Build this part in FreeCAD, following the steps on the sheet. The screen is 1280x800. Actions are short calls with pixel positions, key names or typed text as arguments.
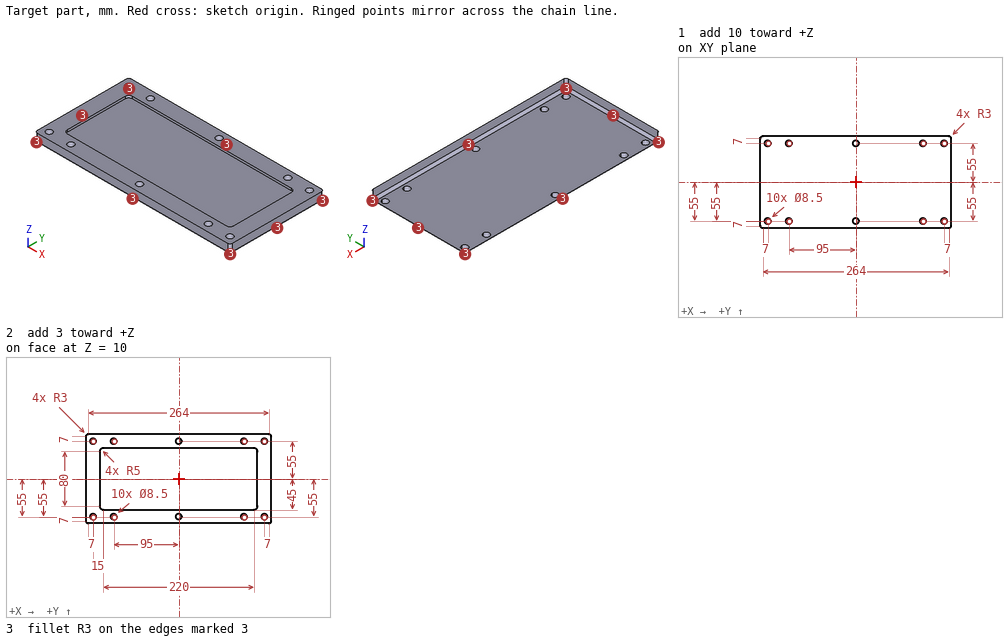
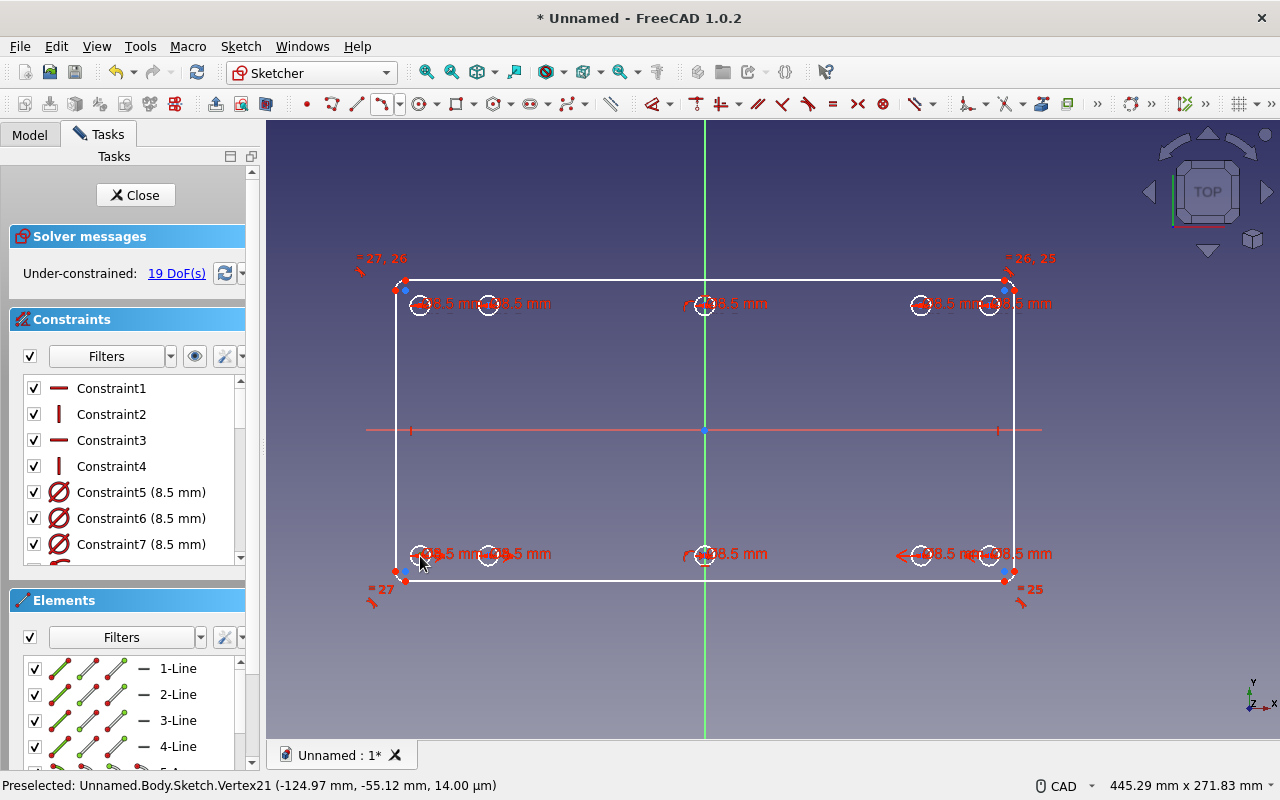
click(420, 306)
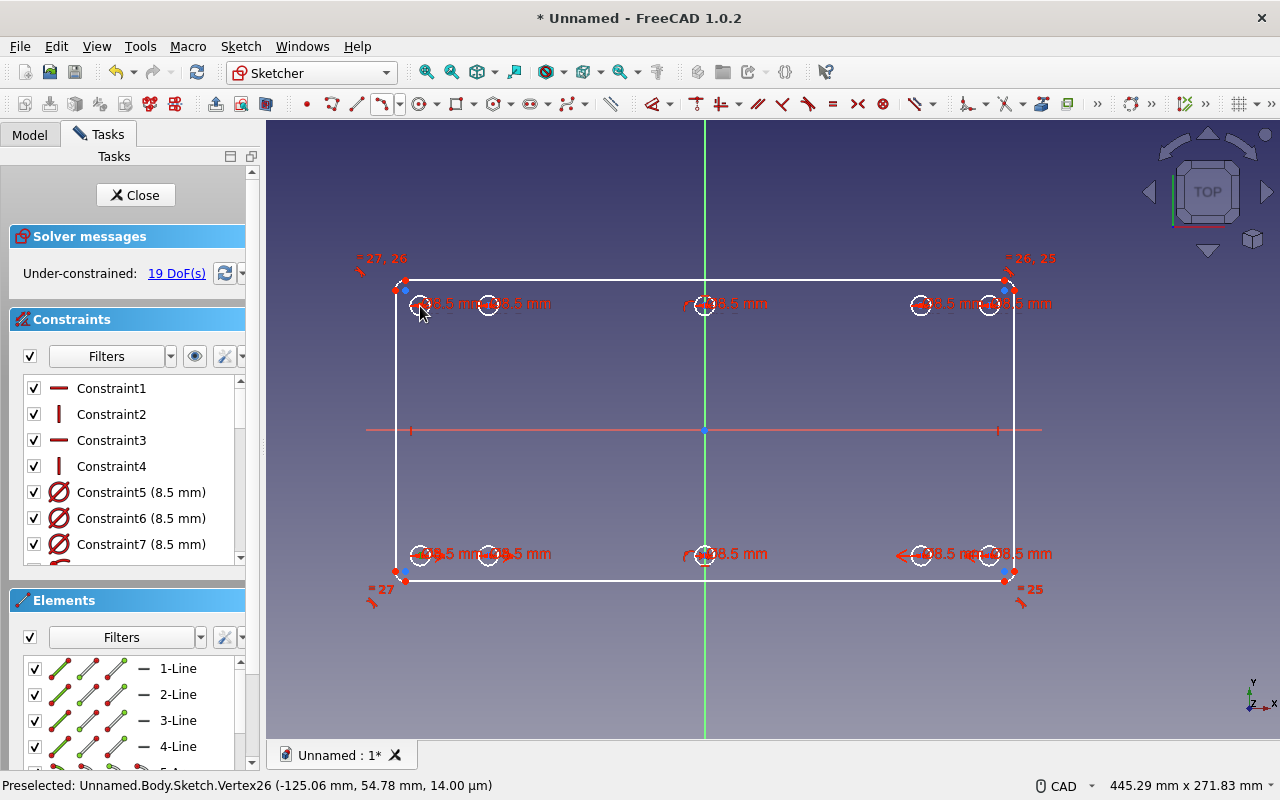
click(470, 430)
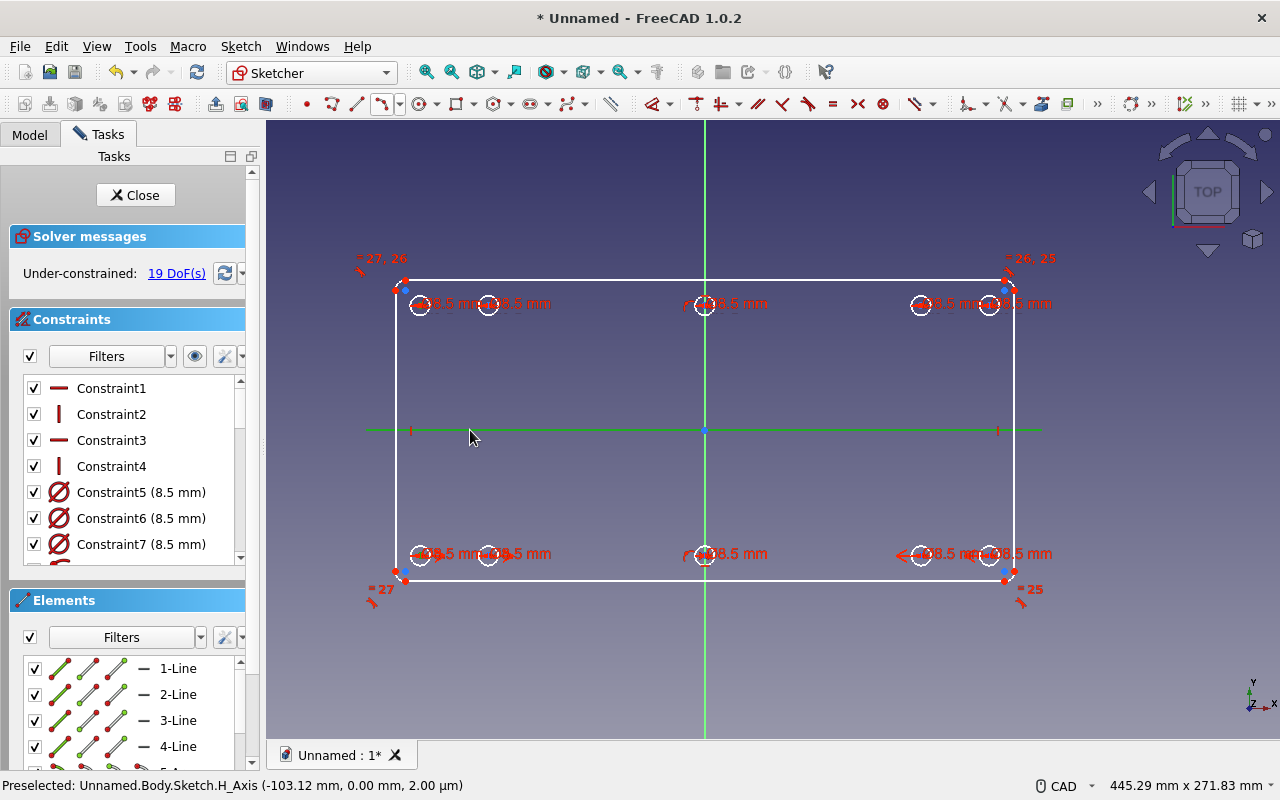
click(858, 104)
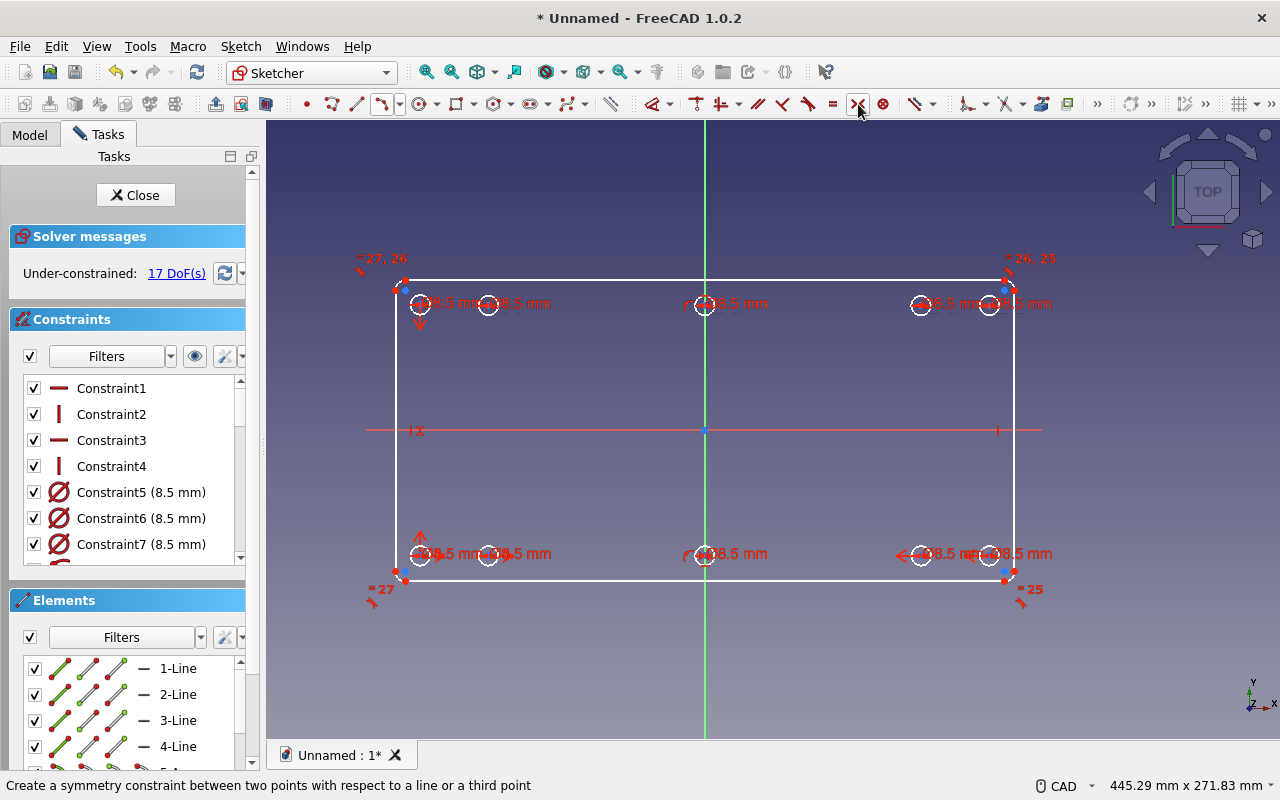
click(488, 556)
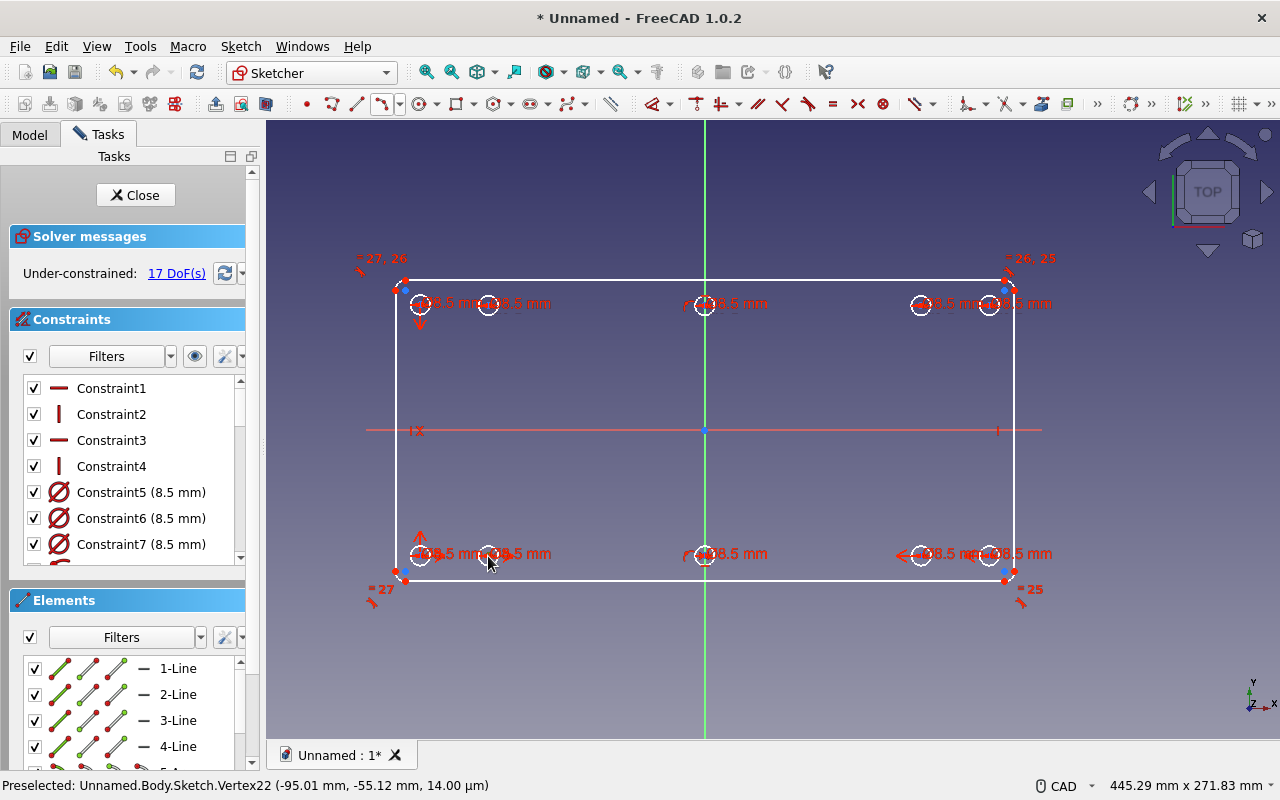
click(488, 306)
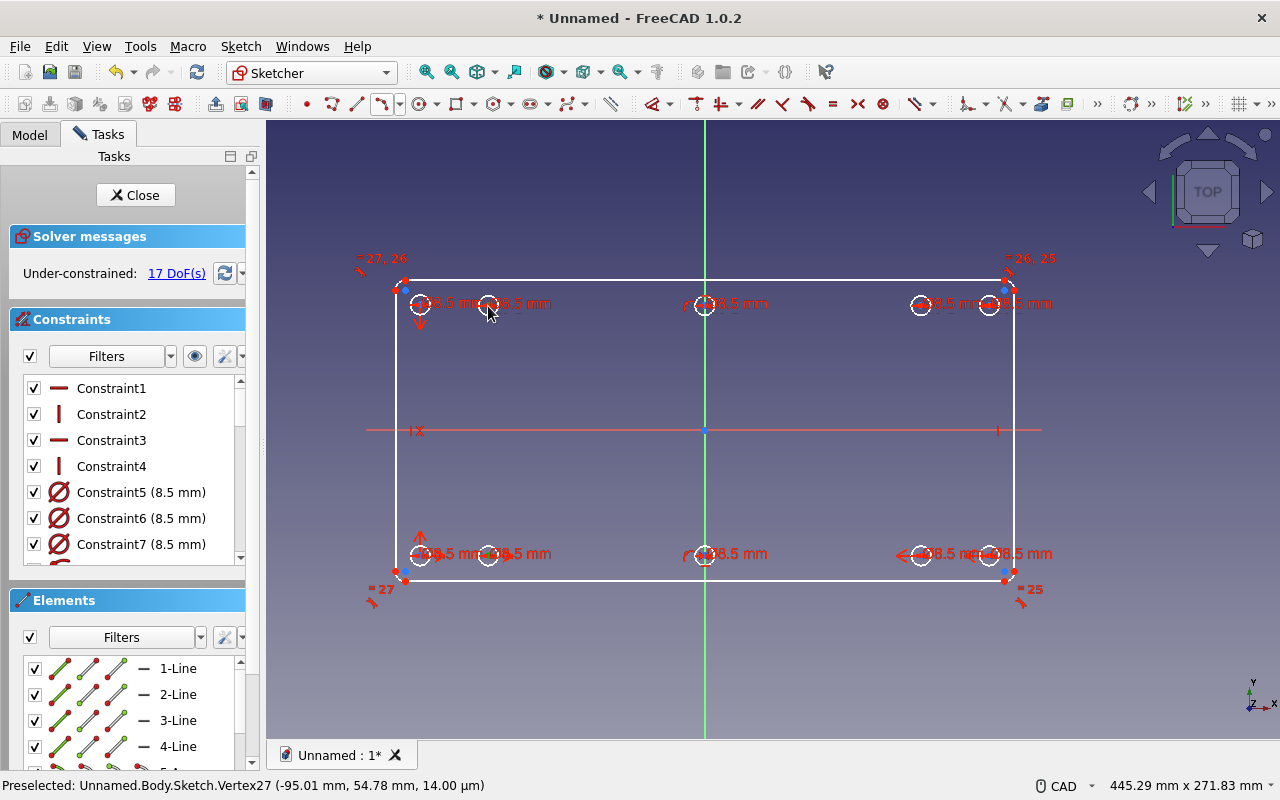
click(470, 430)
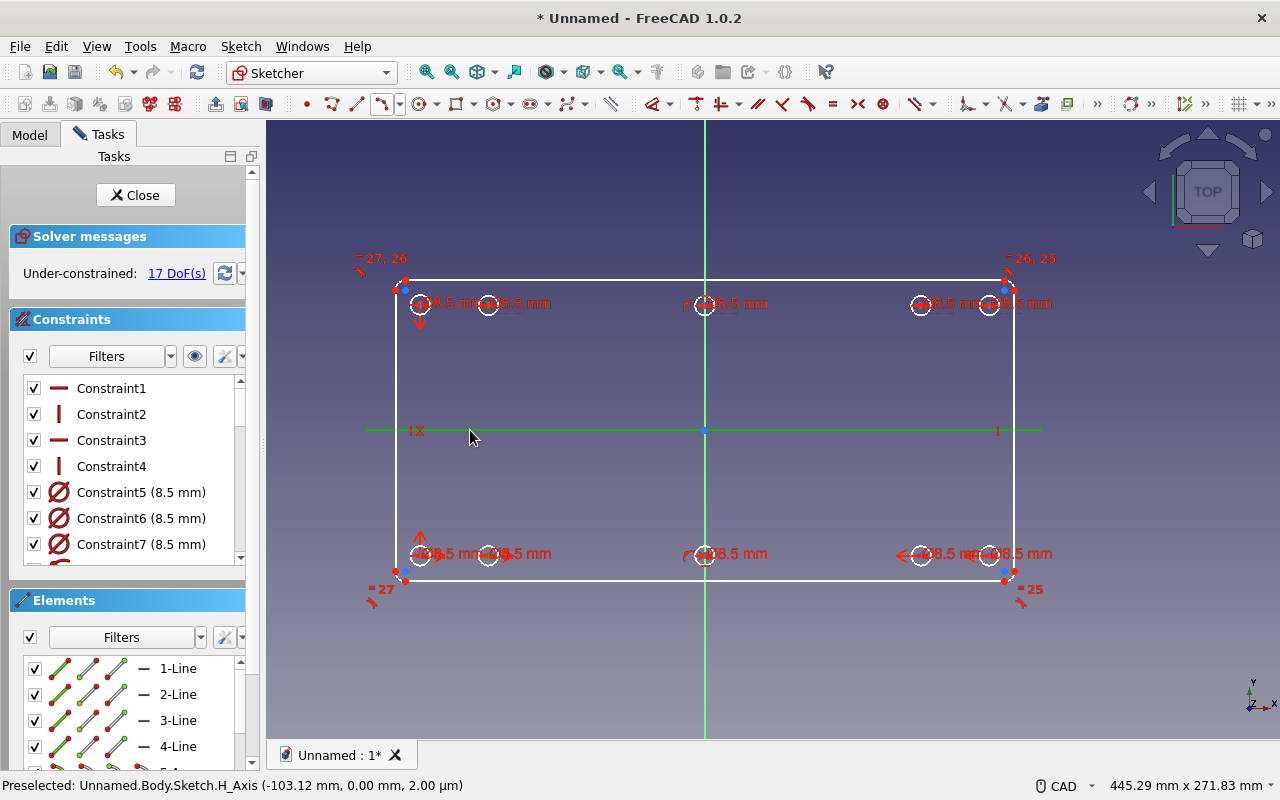
click(858, 104)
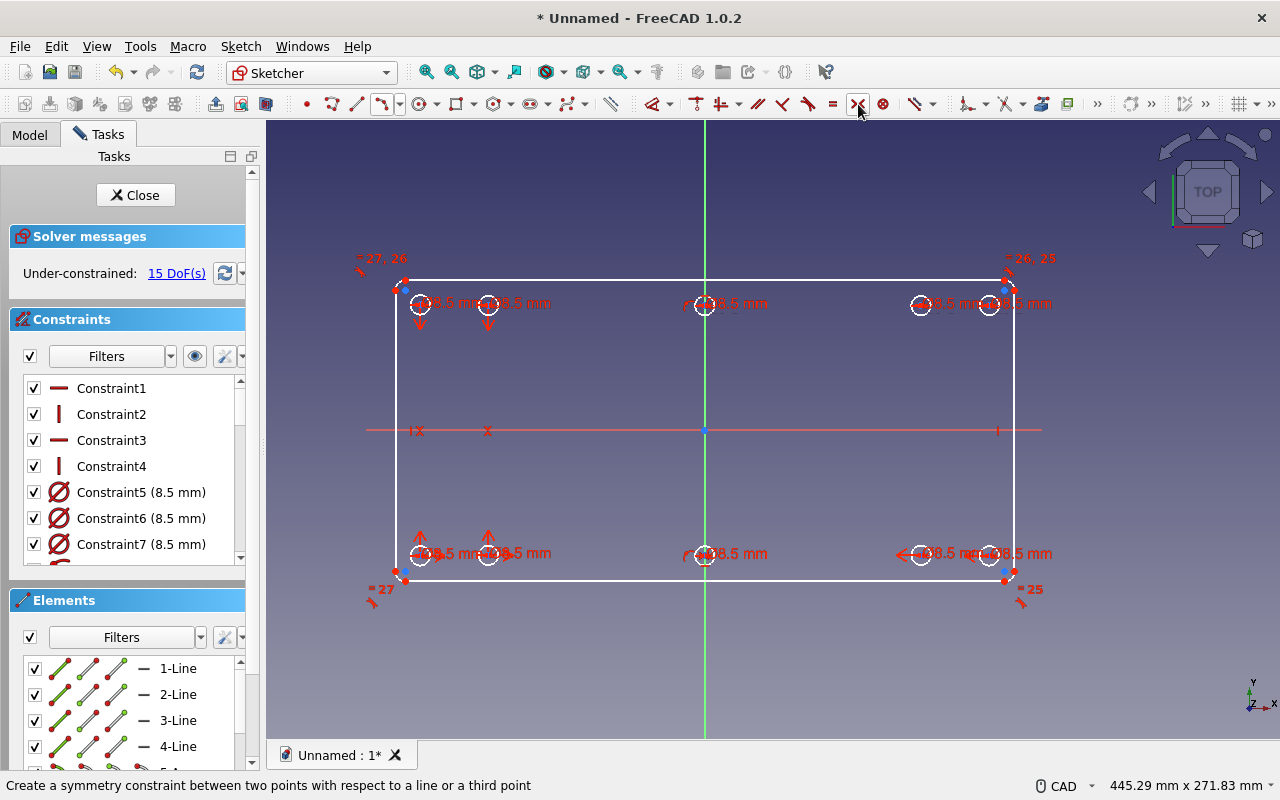
click(921, 555)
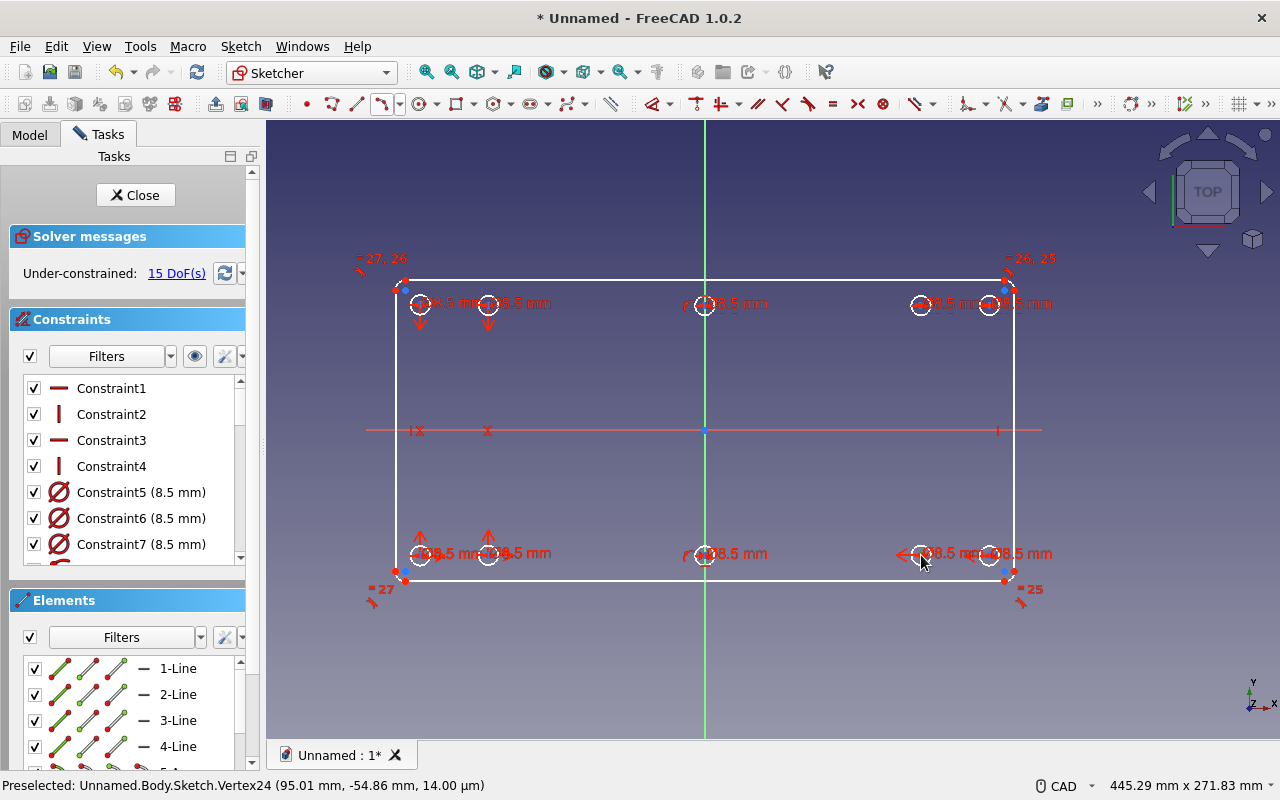
click(921, 306)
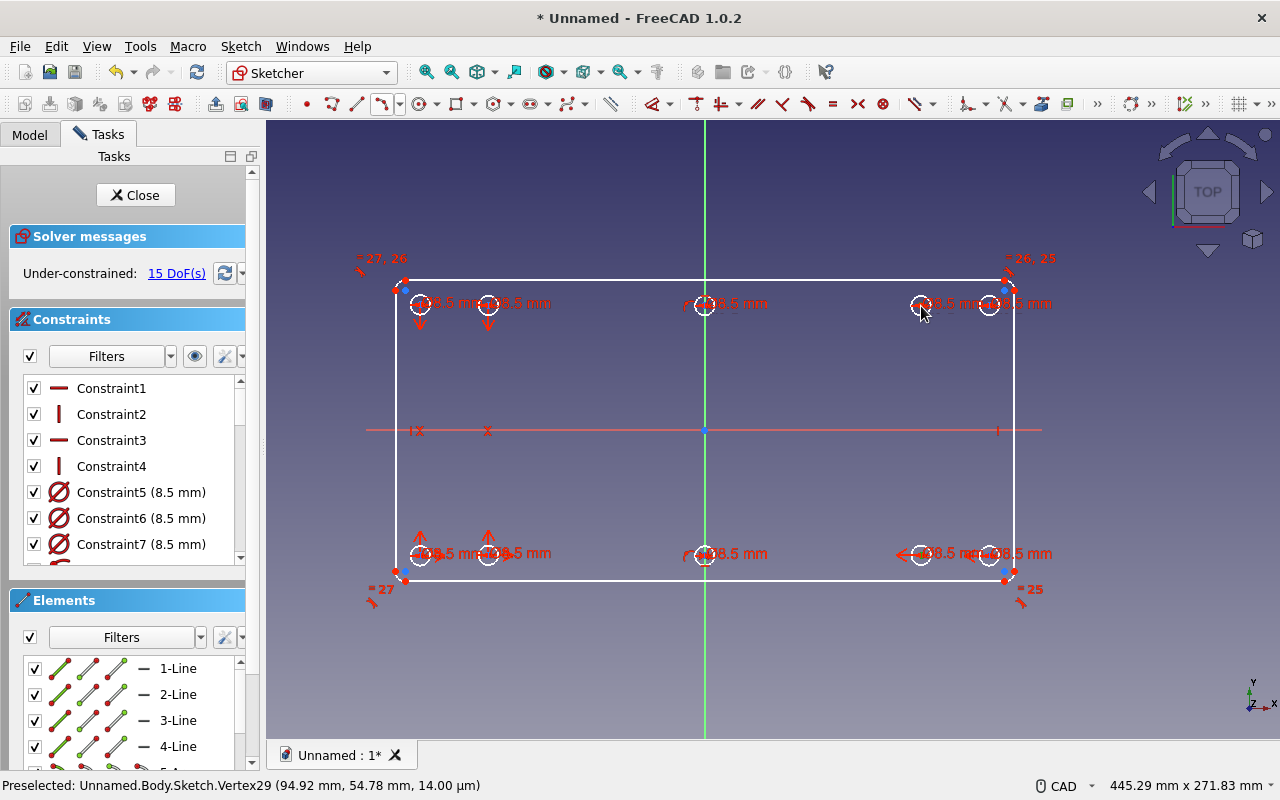
click(470, 430)